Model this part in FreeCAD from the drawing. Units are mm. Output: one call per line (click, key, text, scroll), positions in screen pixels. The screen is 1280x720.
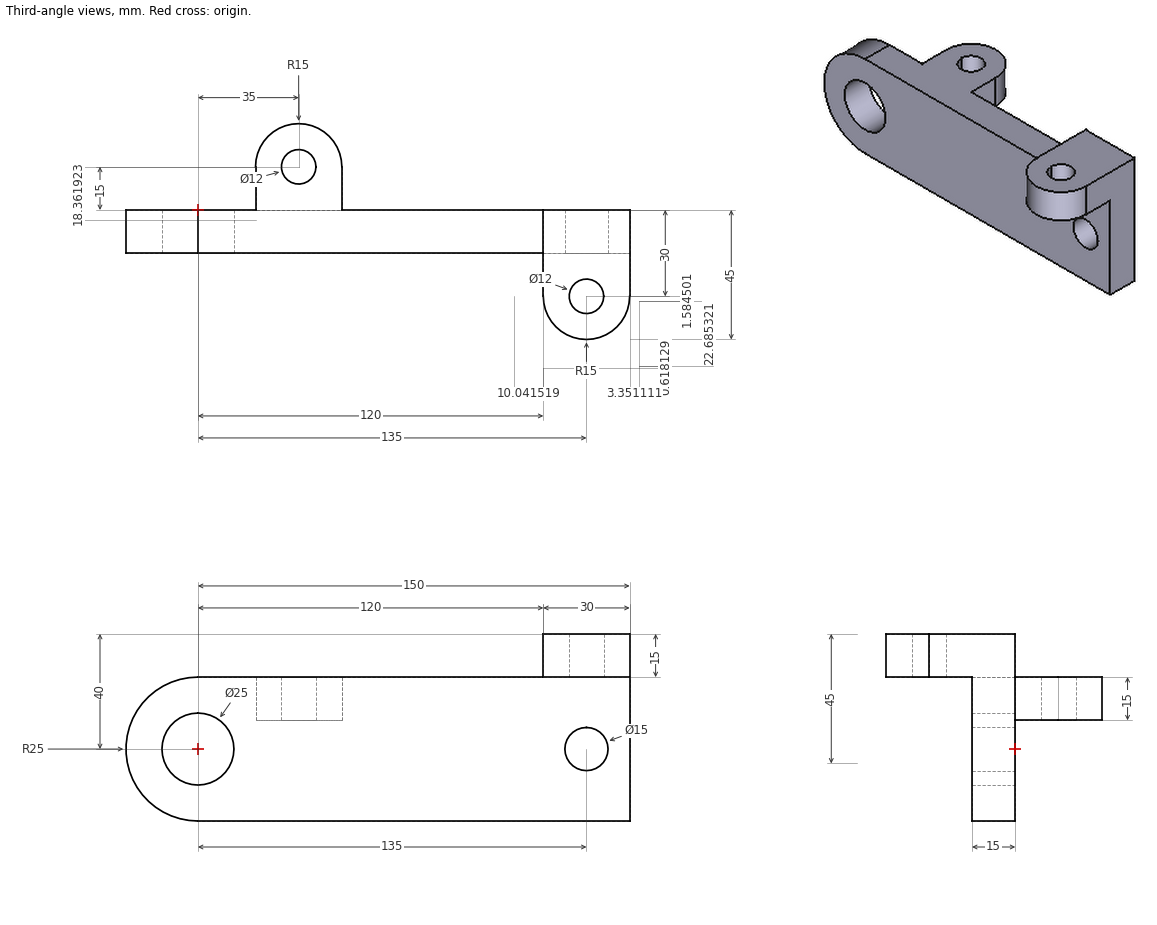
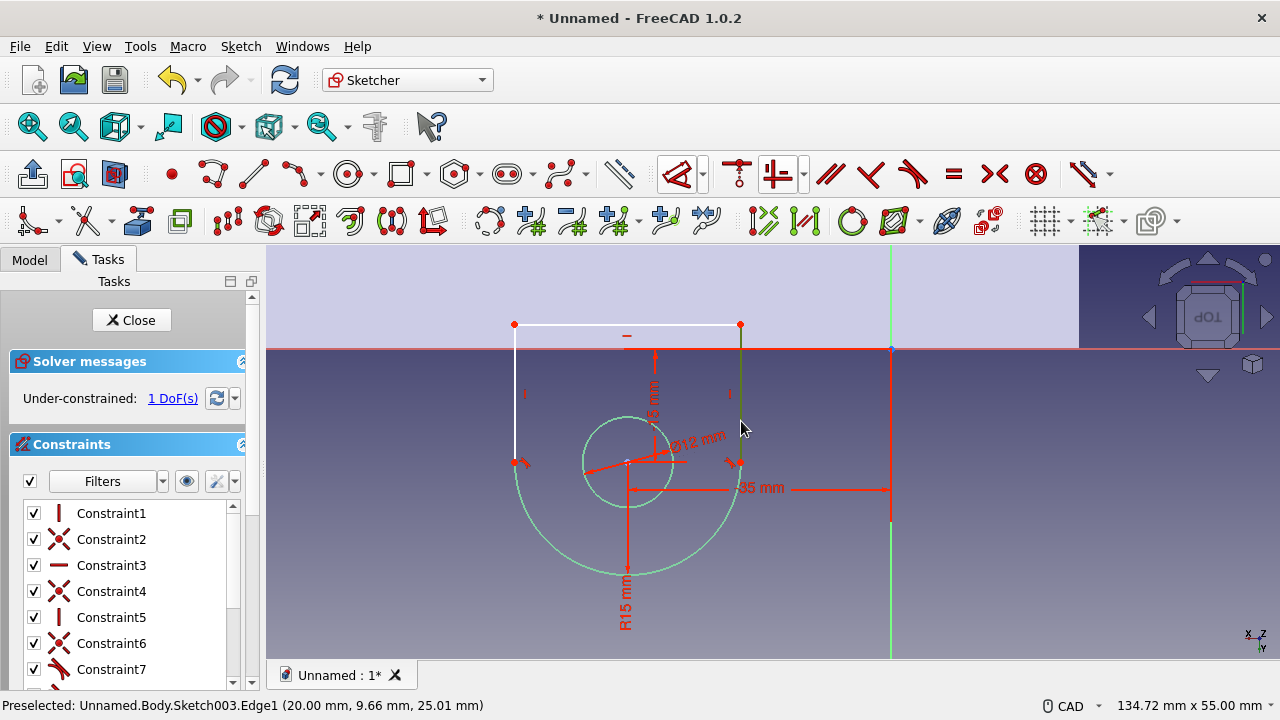
click(702, 174)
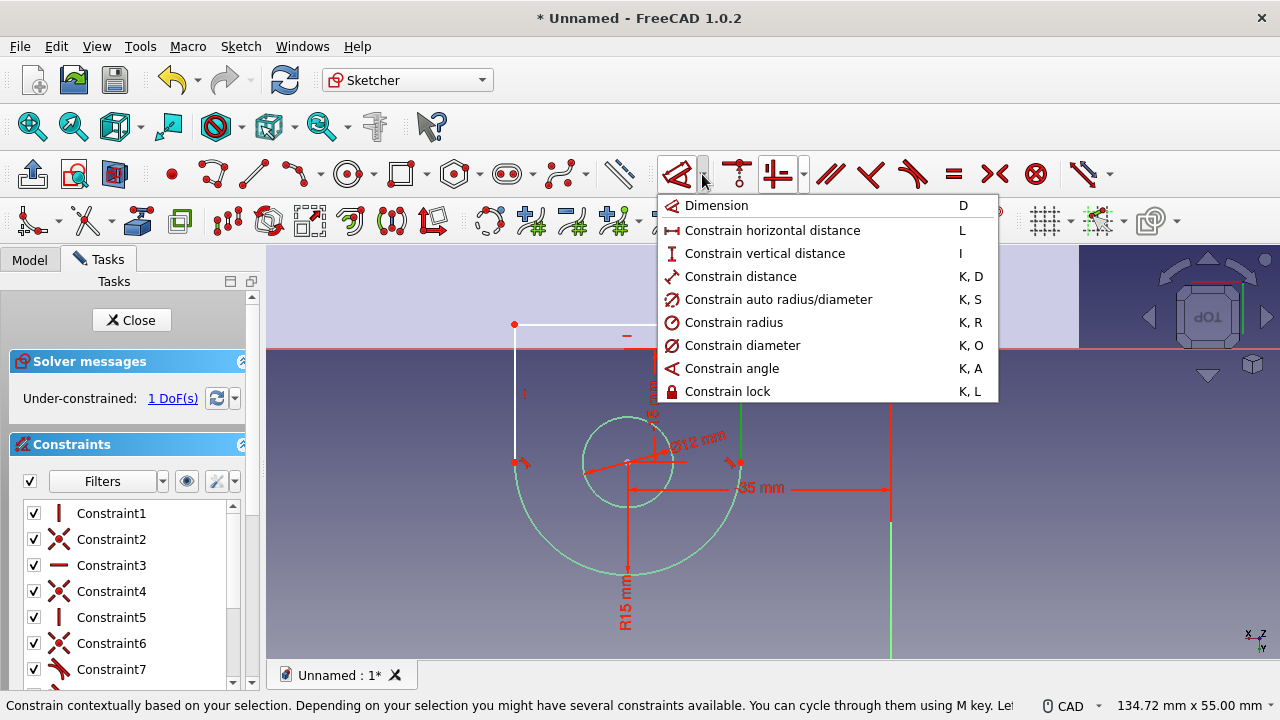
click(828, 254)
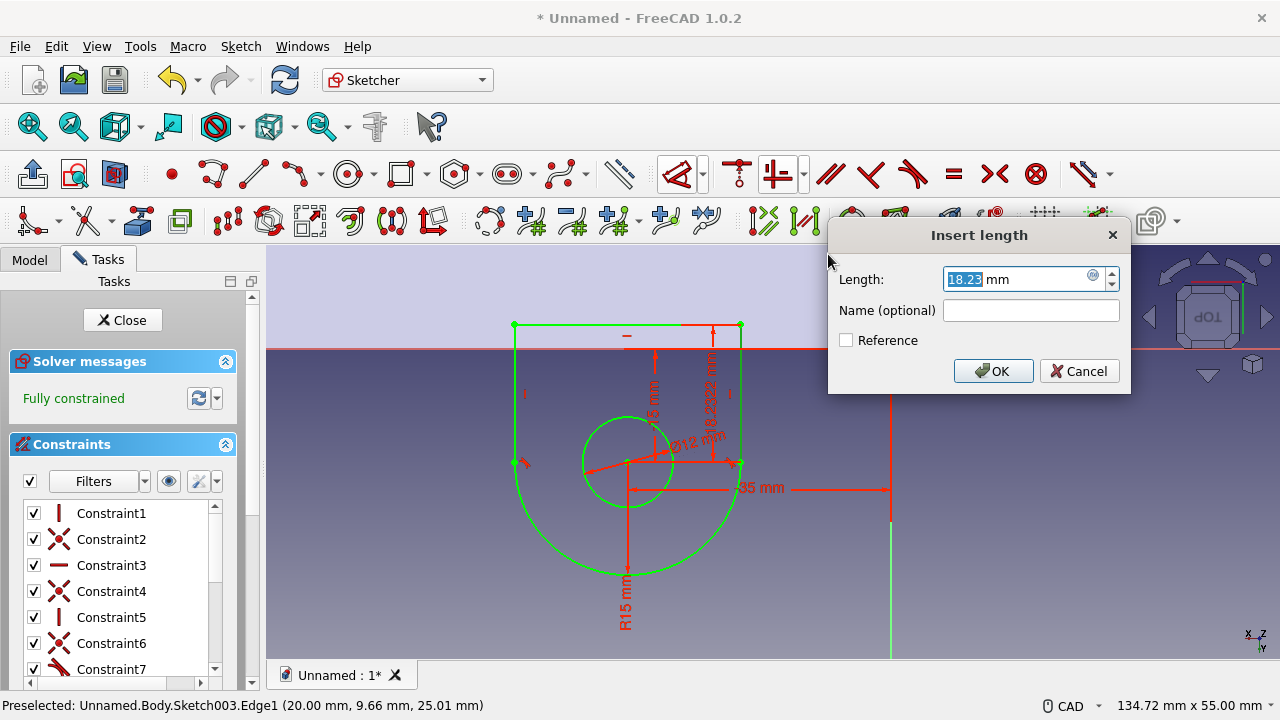
text(18.361923)
key(Return)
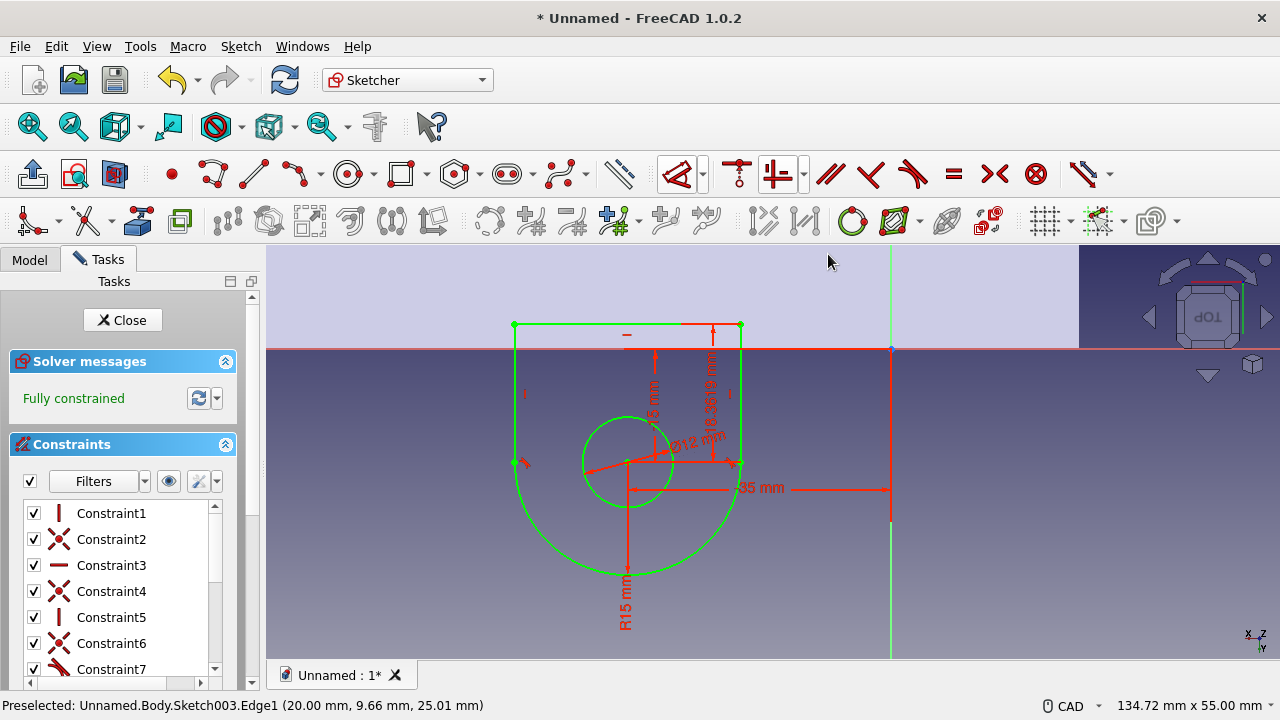
click(123, 320)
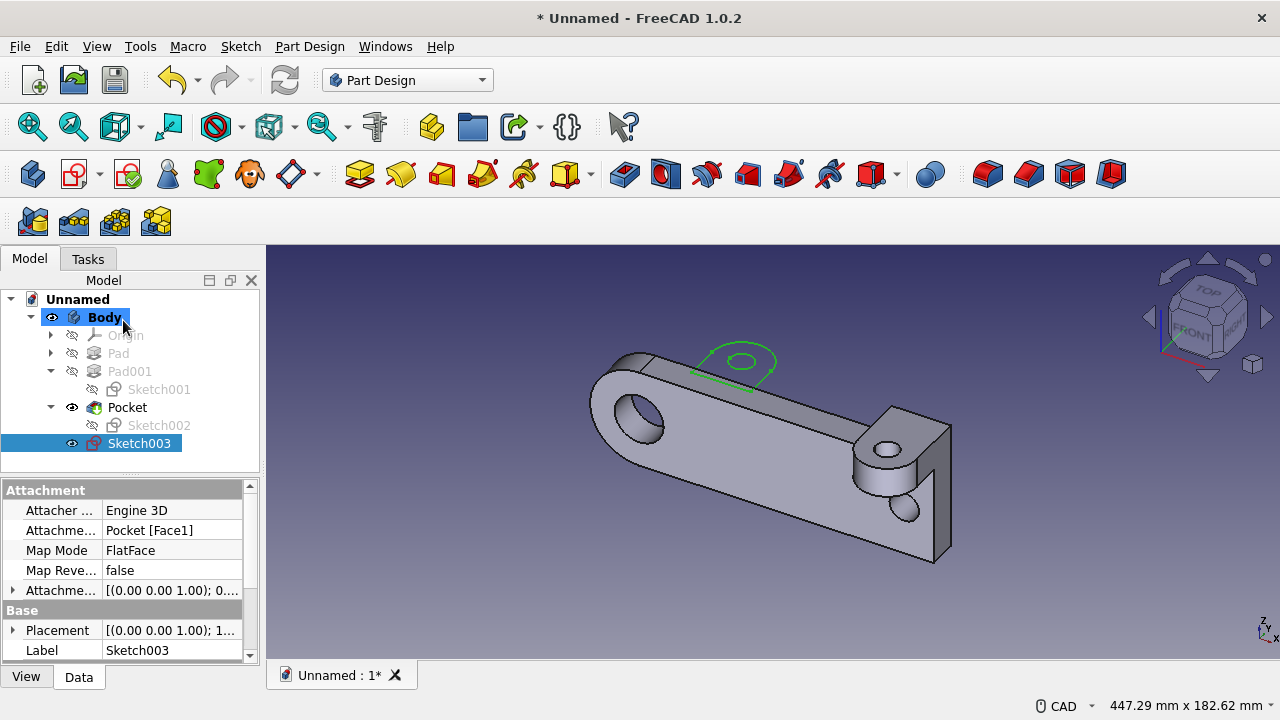
click(360, 174)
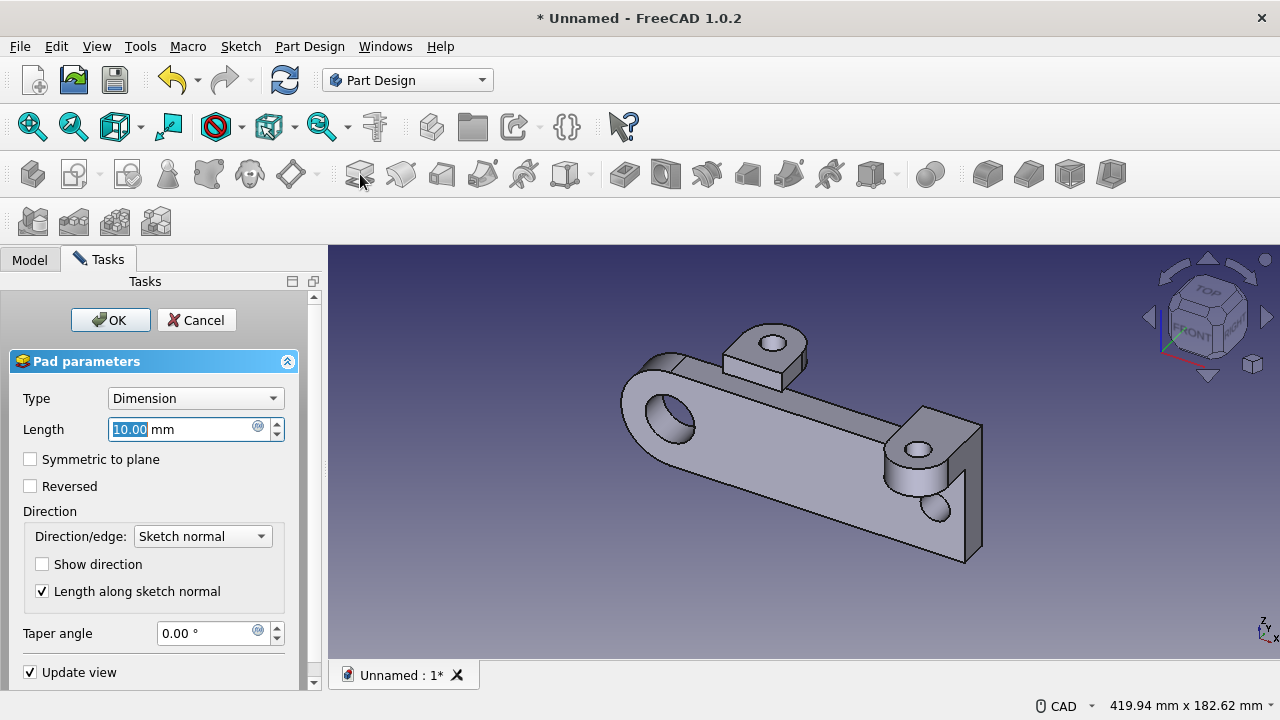
text(15)
key(Tab)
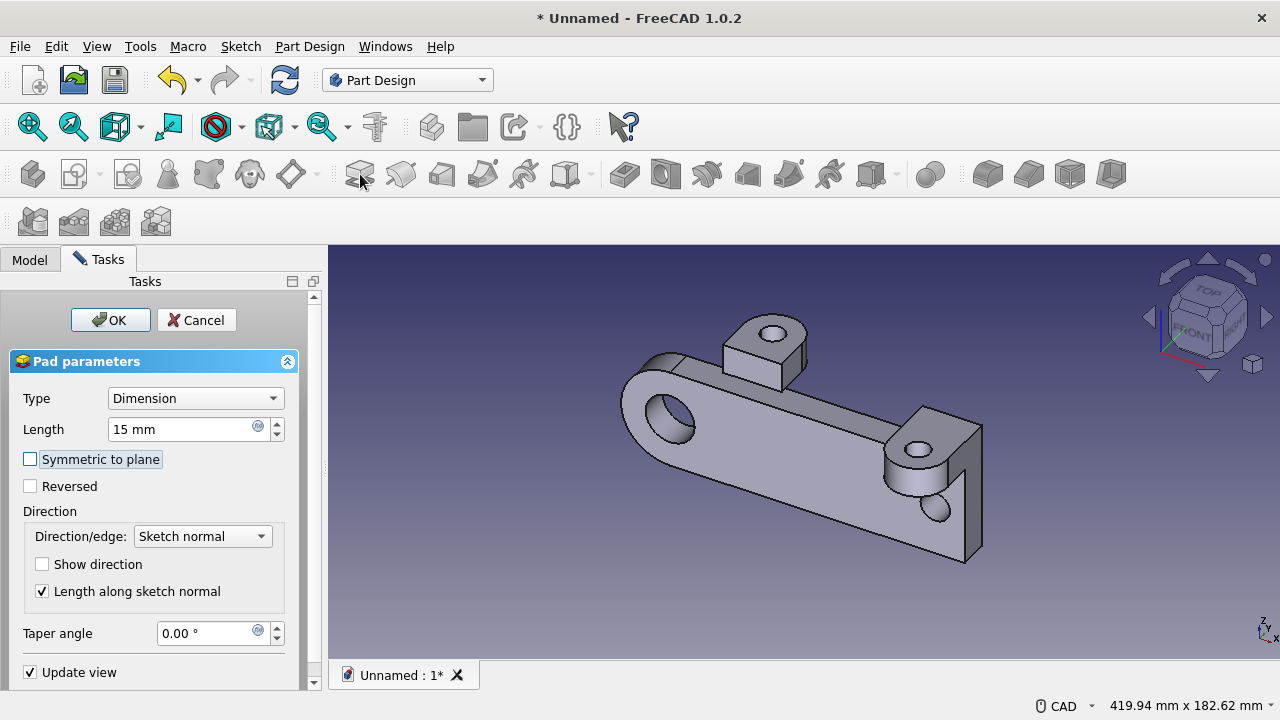
click(31, 486)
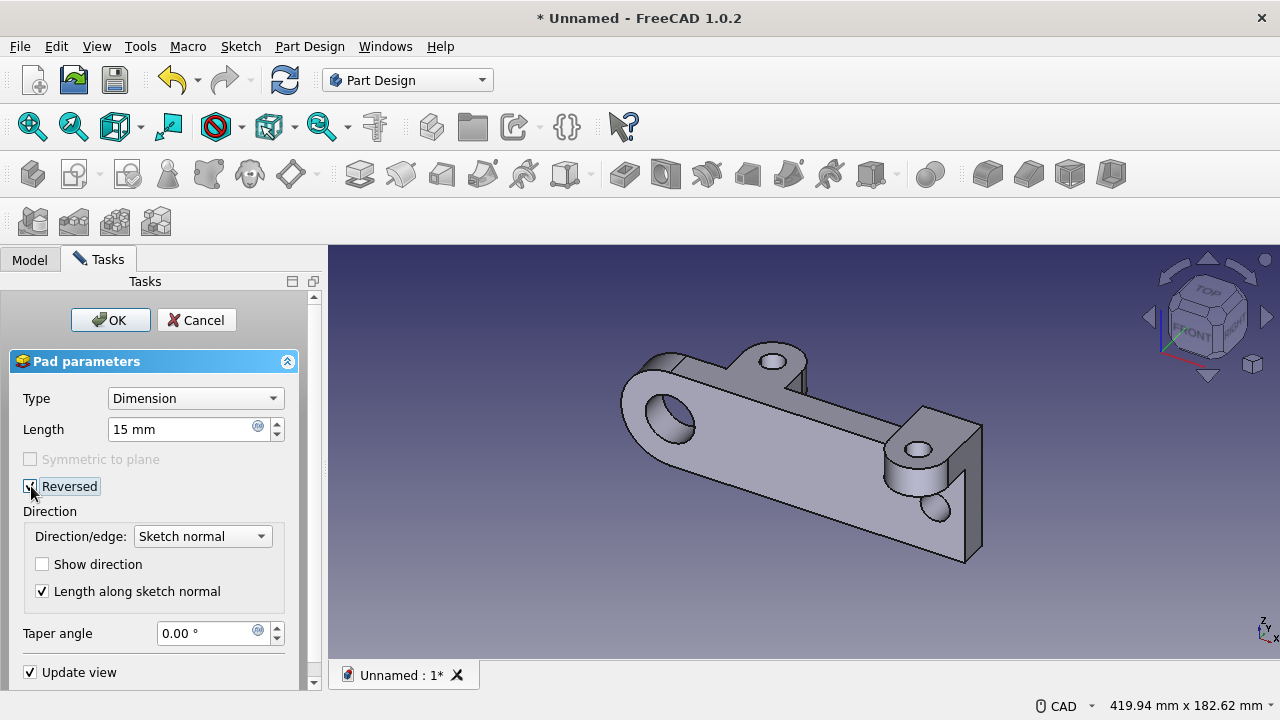
click(111, 320)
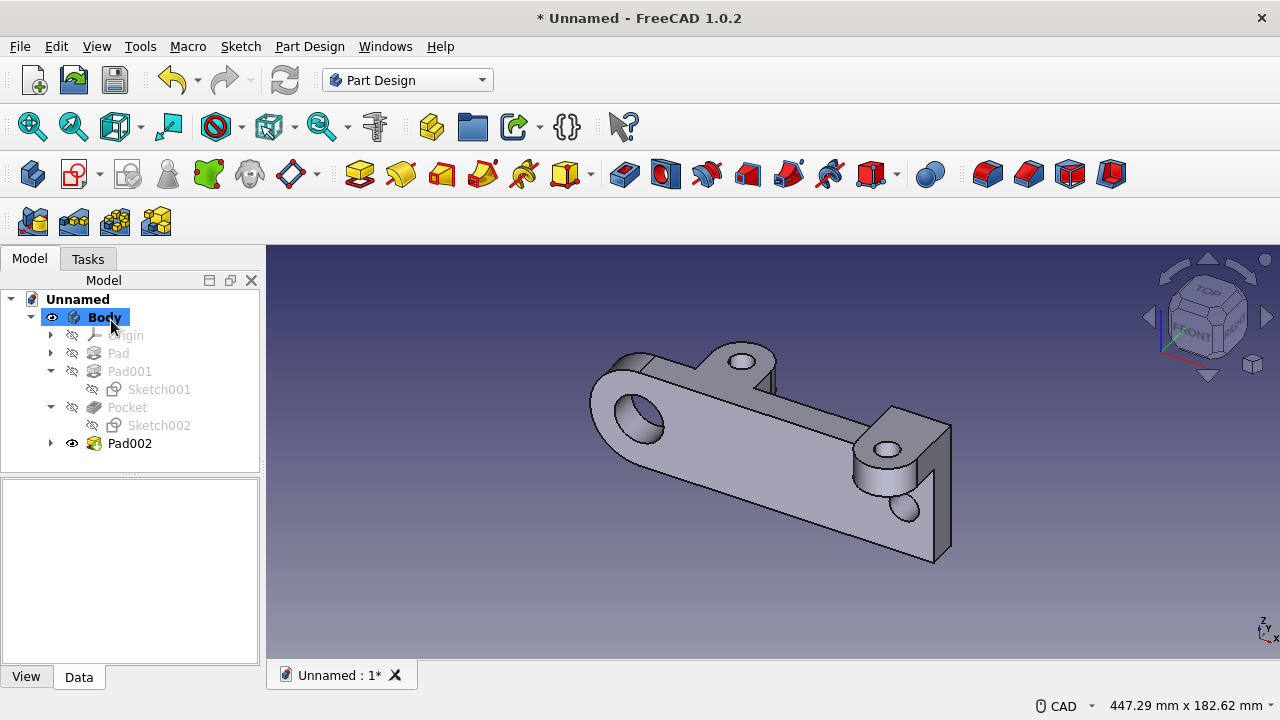
key(0)